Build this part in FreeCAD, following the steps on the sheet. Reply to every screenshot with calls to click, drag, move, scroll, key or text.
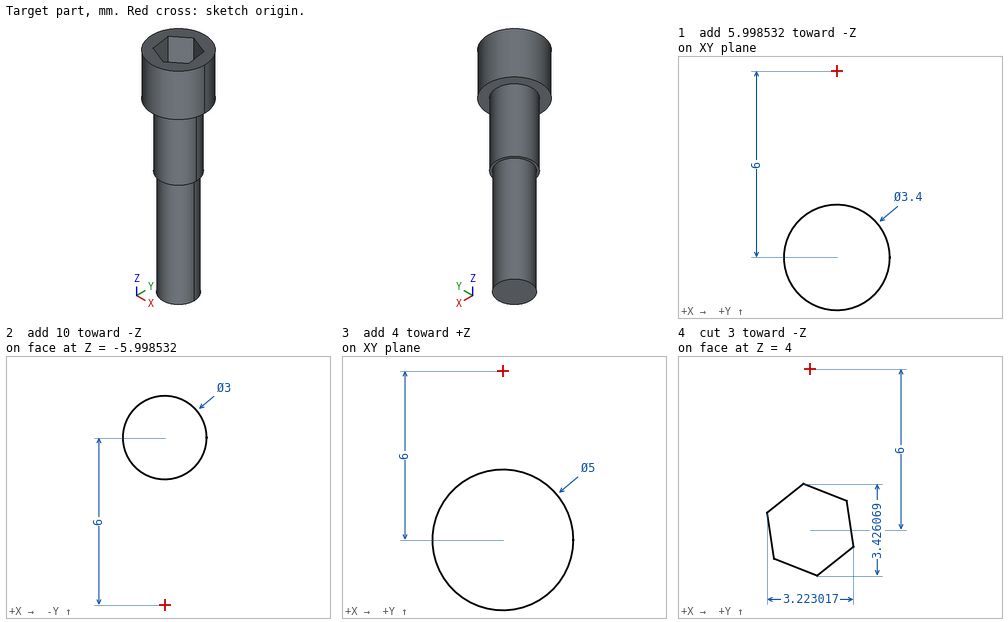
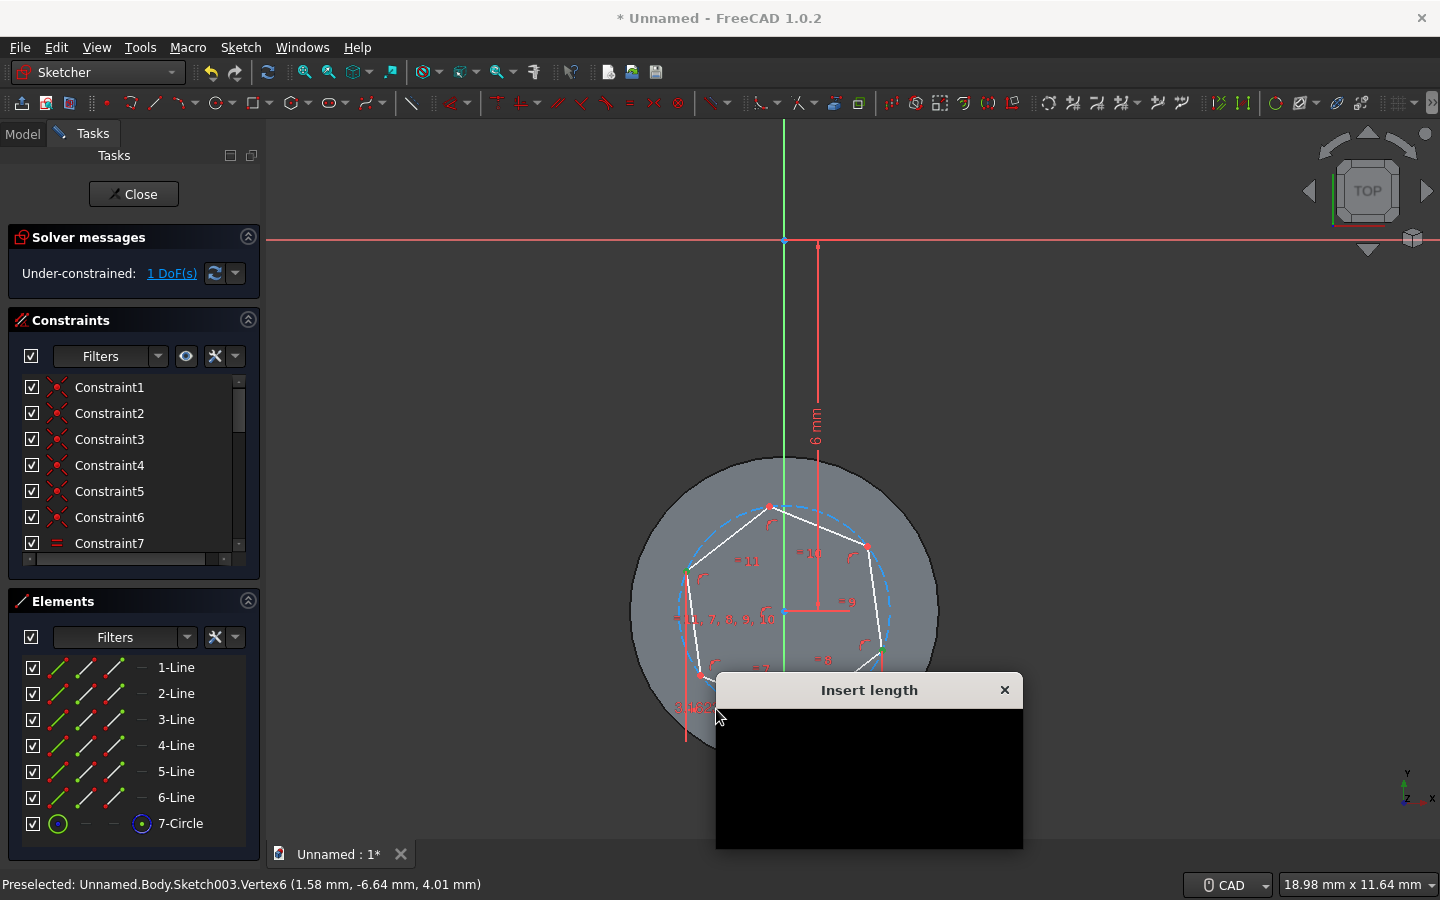
text(3.223017)
key(Return)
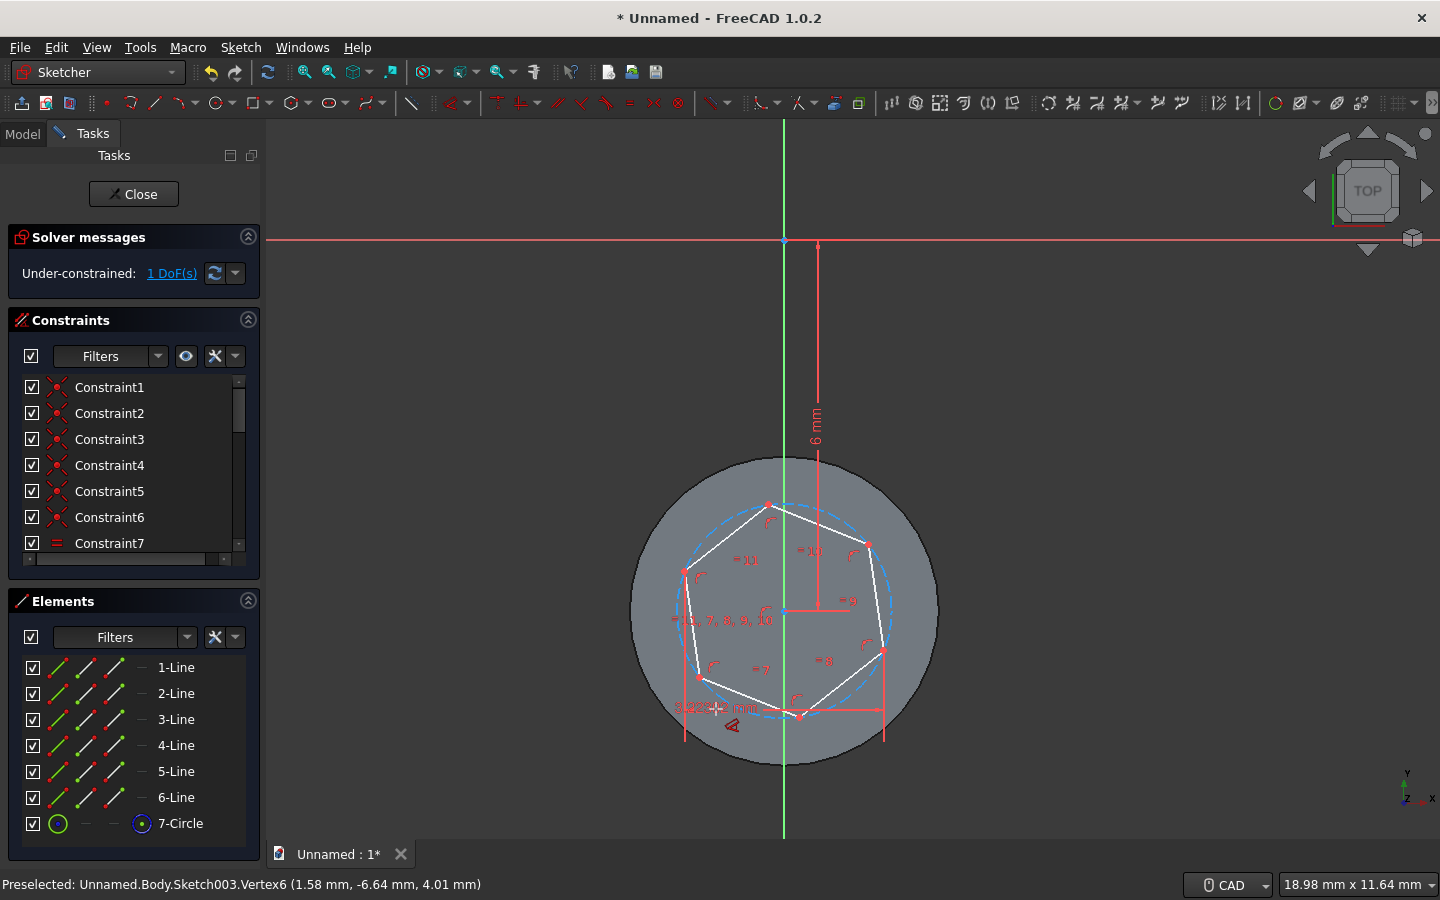
click(800, 717)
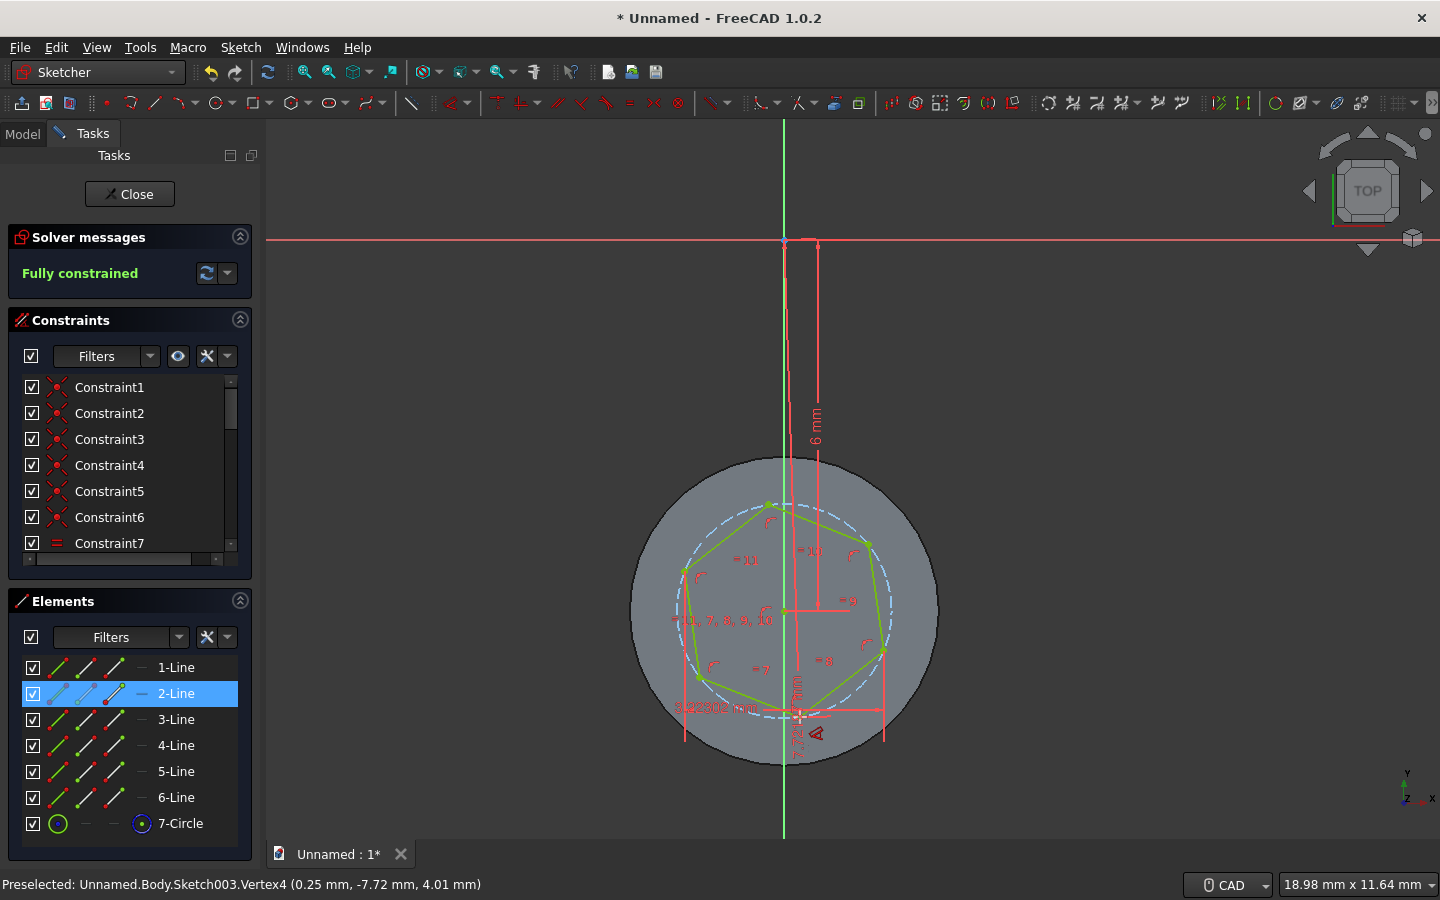
click(769, 505)
click(834, 611)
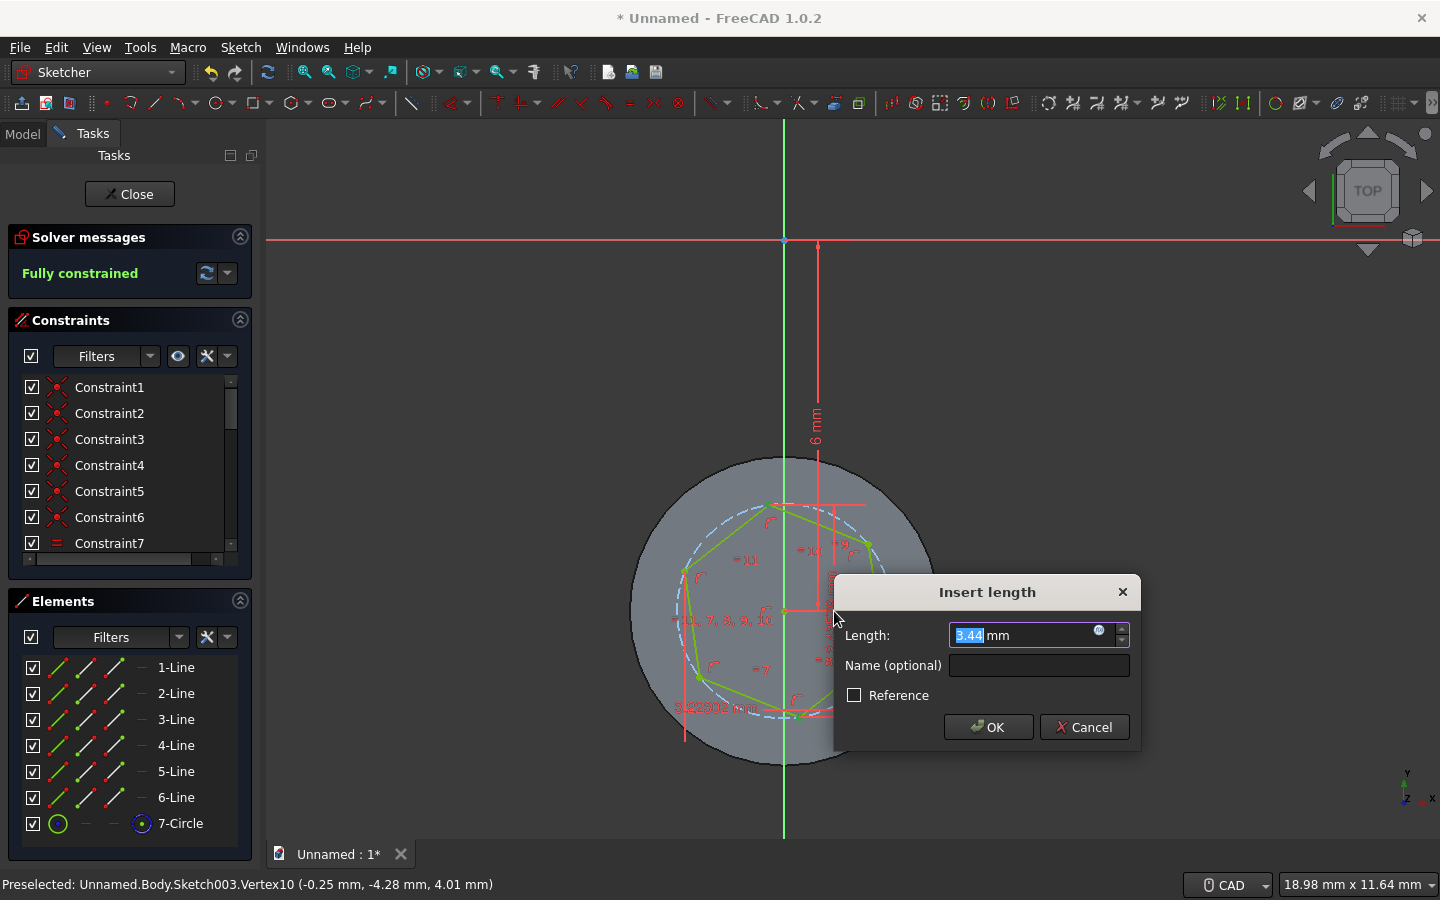
text(3.426069)
key(Return)
key(Escape)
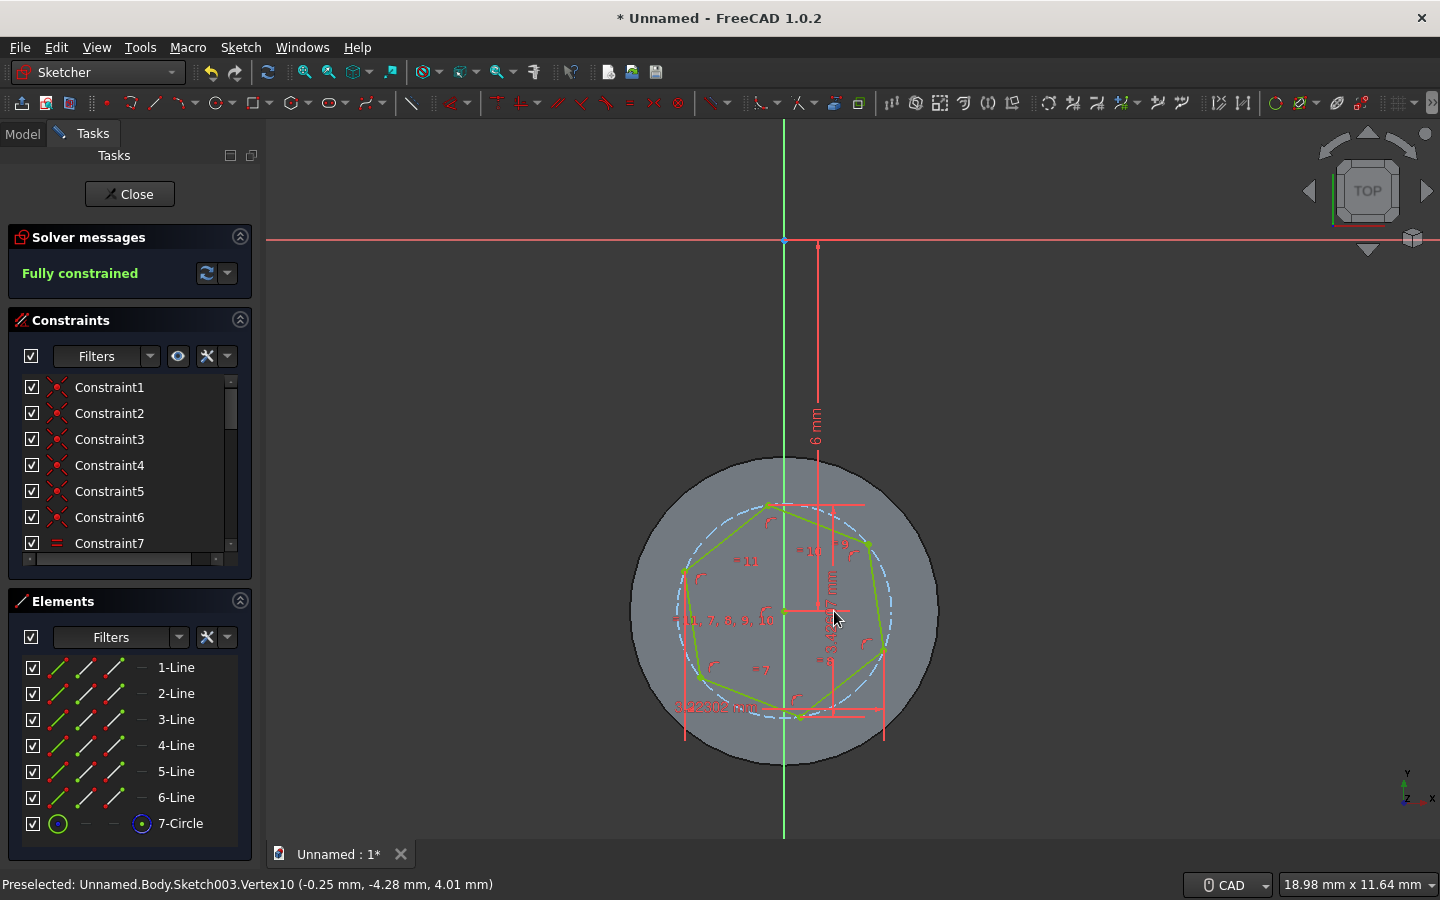
click(130, 194)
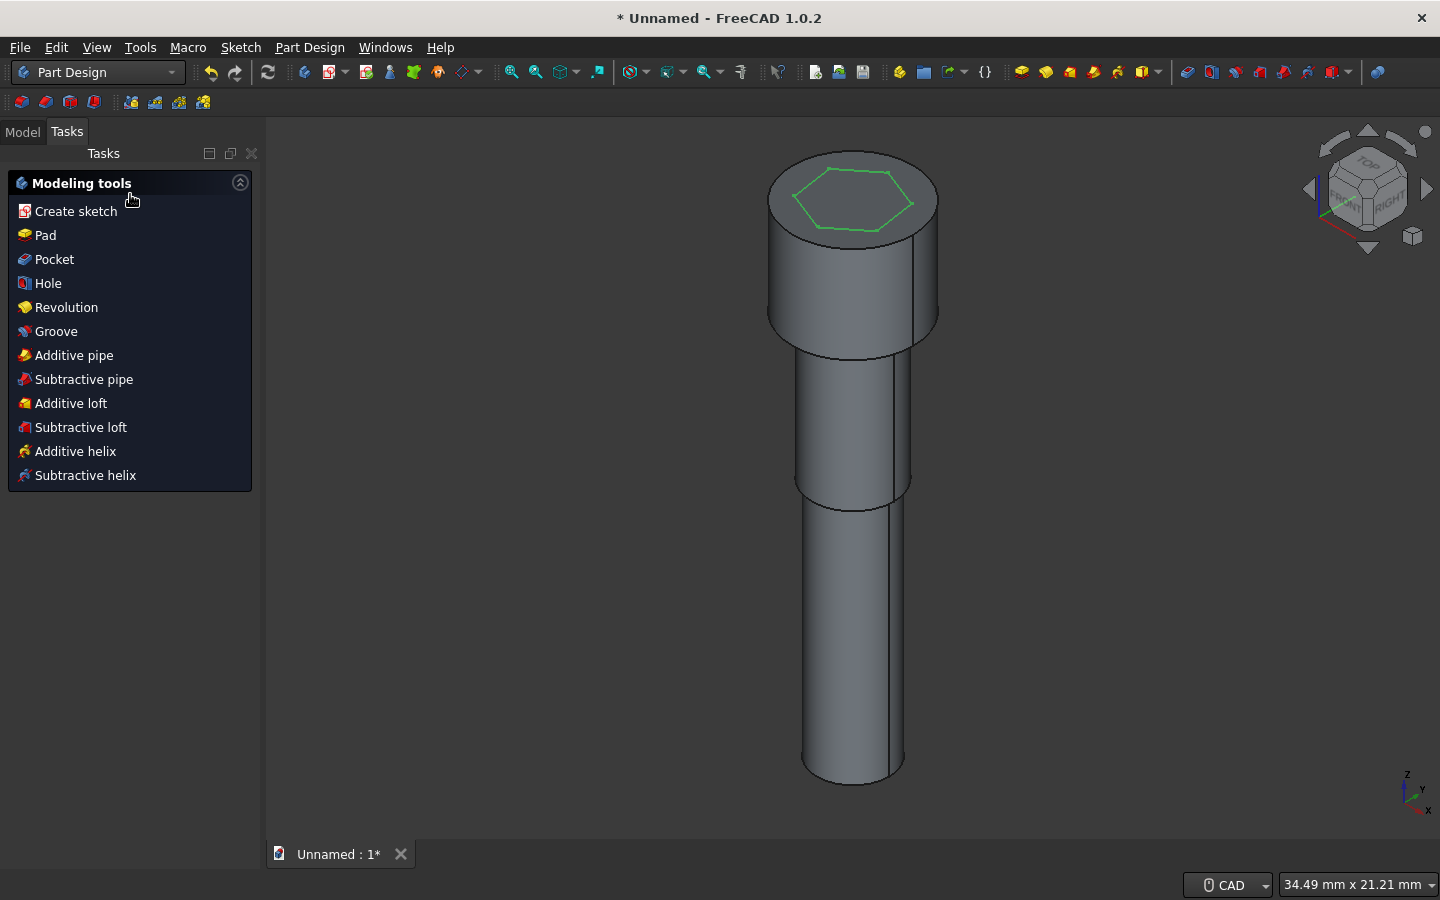
click(1188, 72)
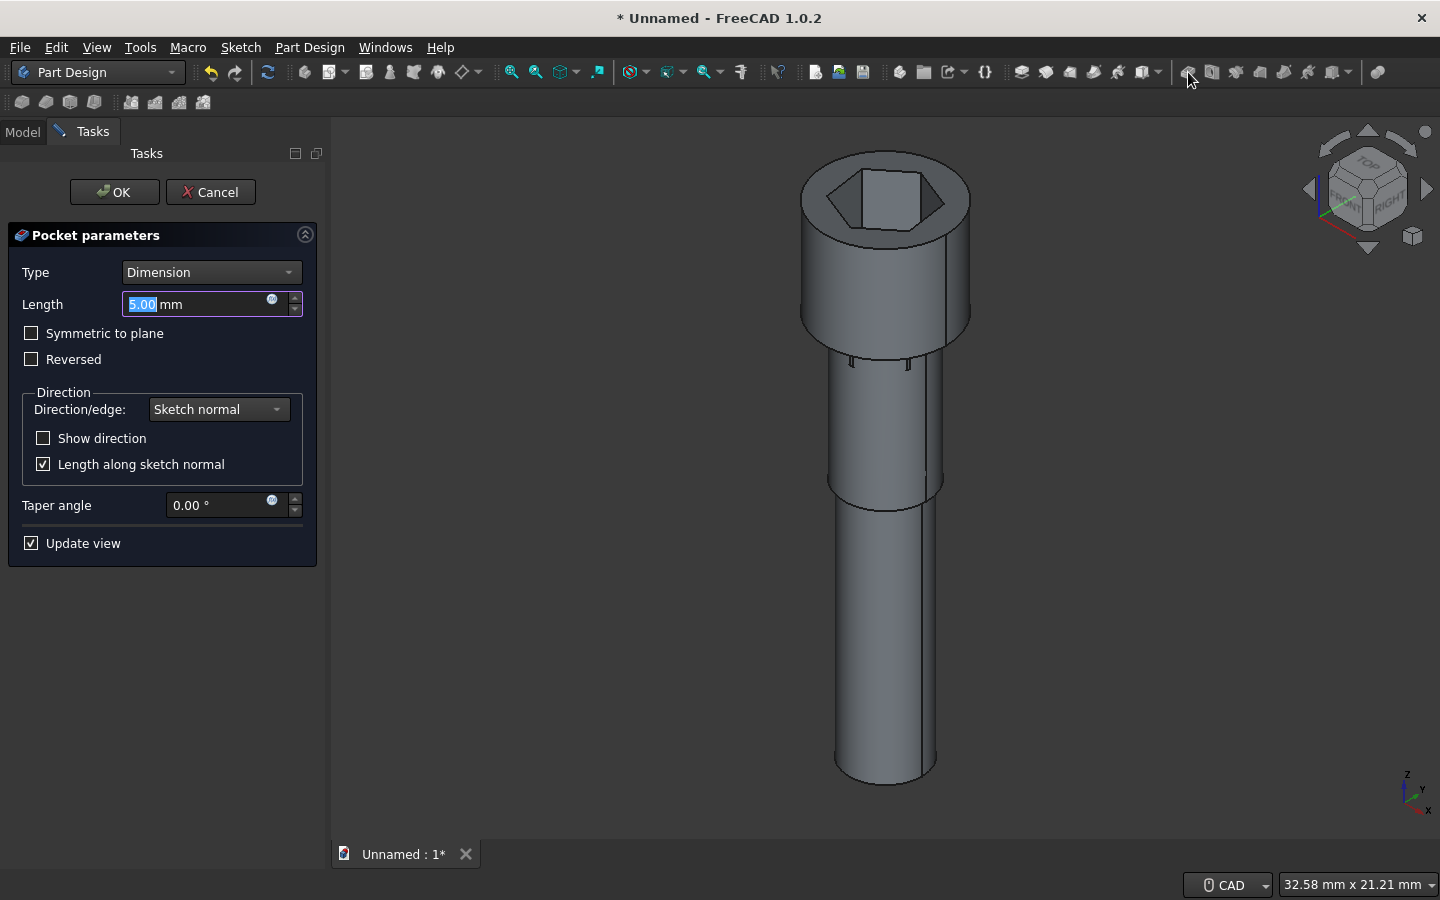
text(3)
key(Tab)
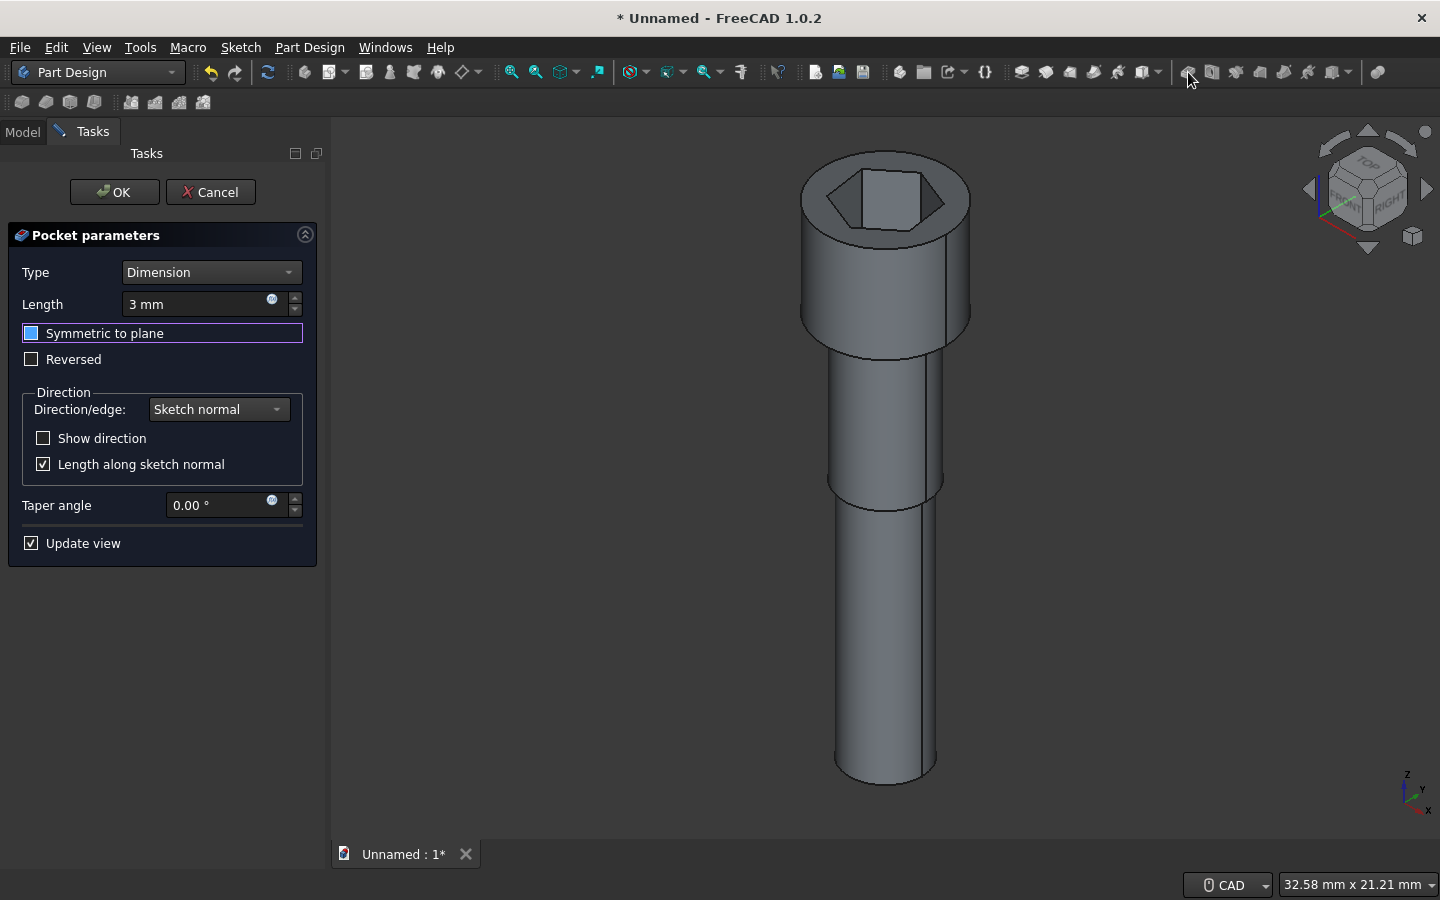
click(115, 192)